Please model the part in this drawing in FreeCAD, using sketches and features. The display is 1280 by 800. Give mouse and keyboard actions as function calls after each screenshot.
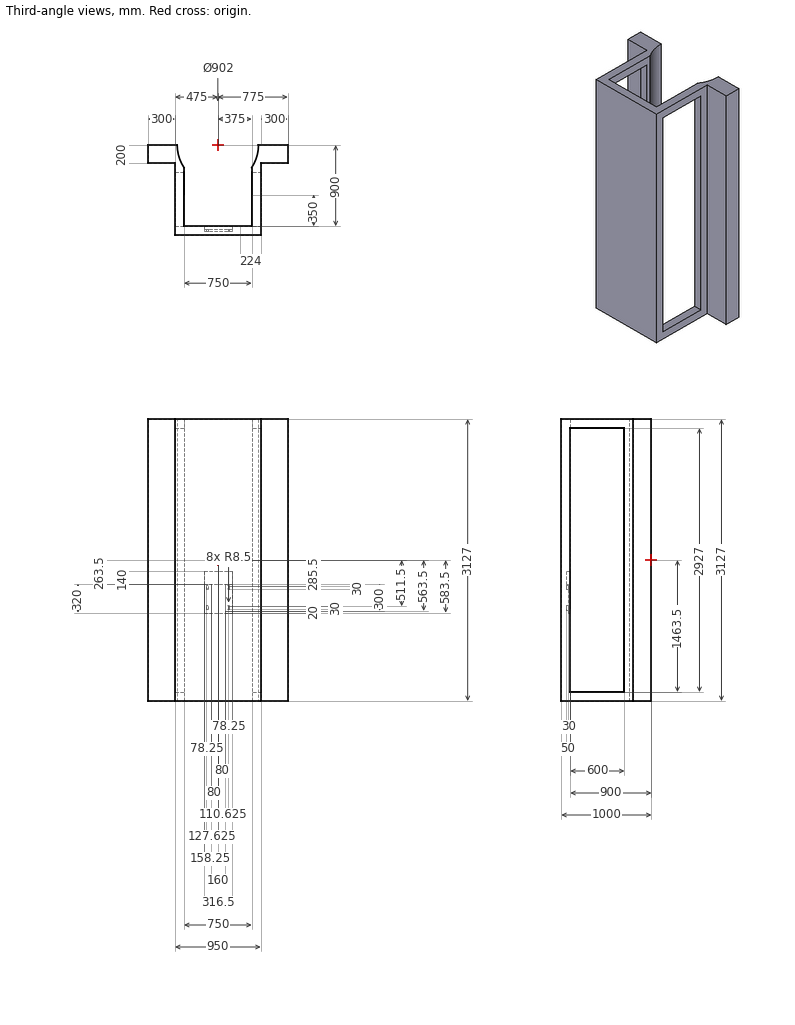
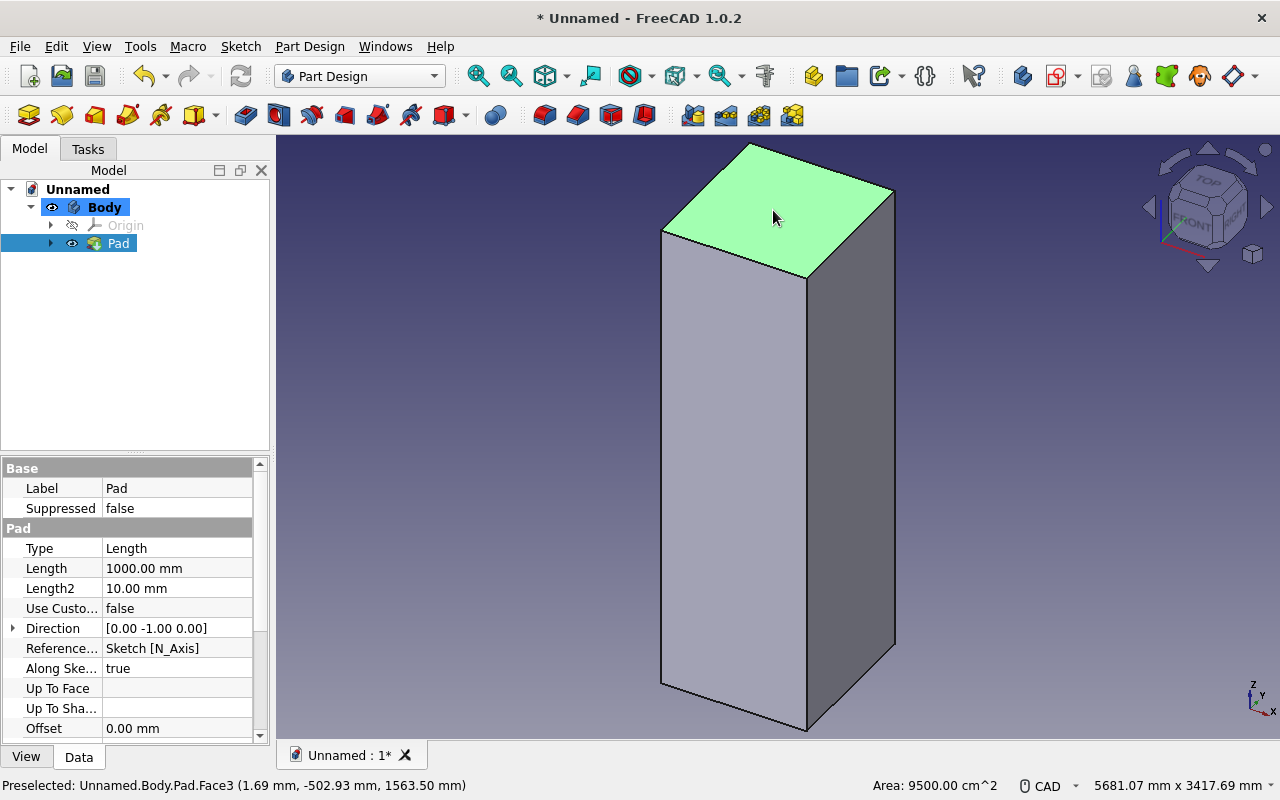
click(1056, 76)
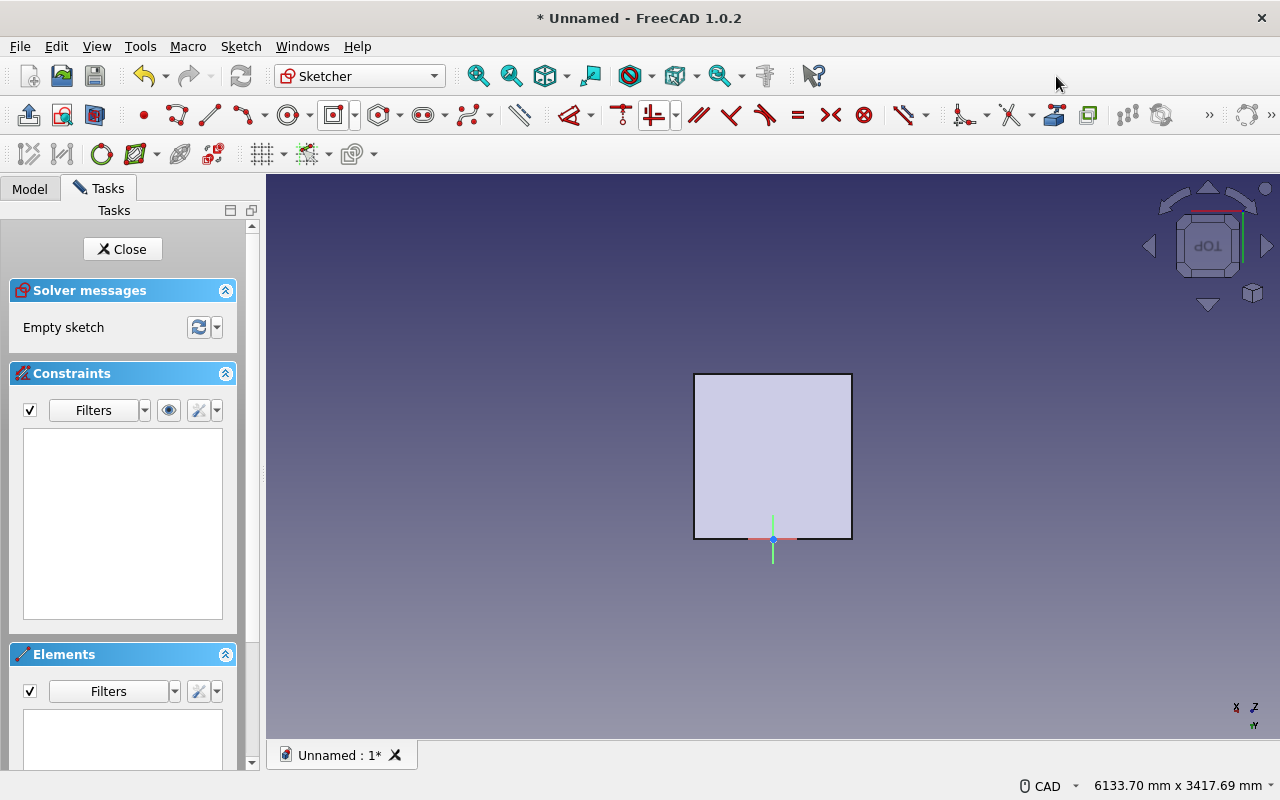
scroll(829, 607, up, 4)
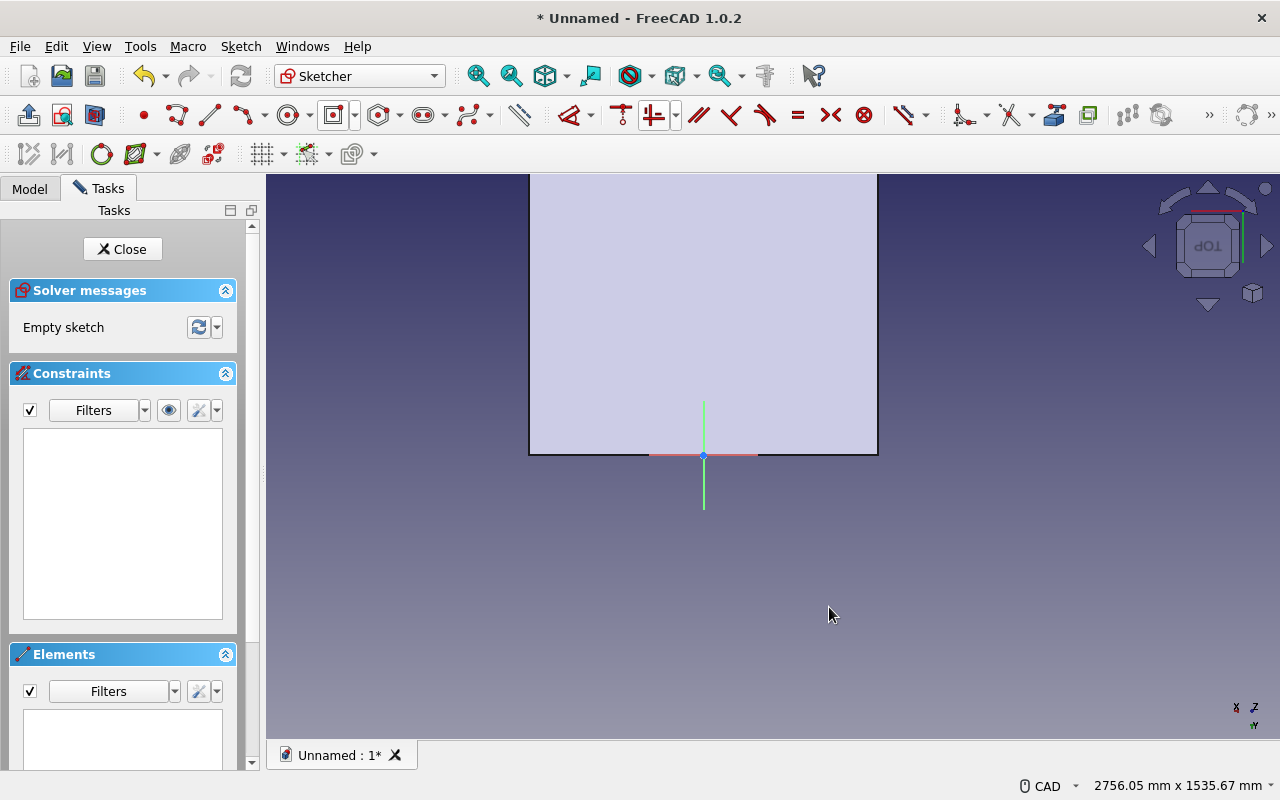
click(288, 116)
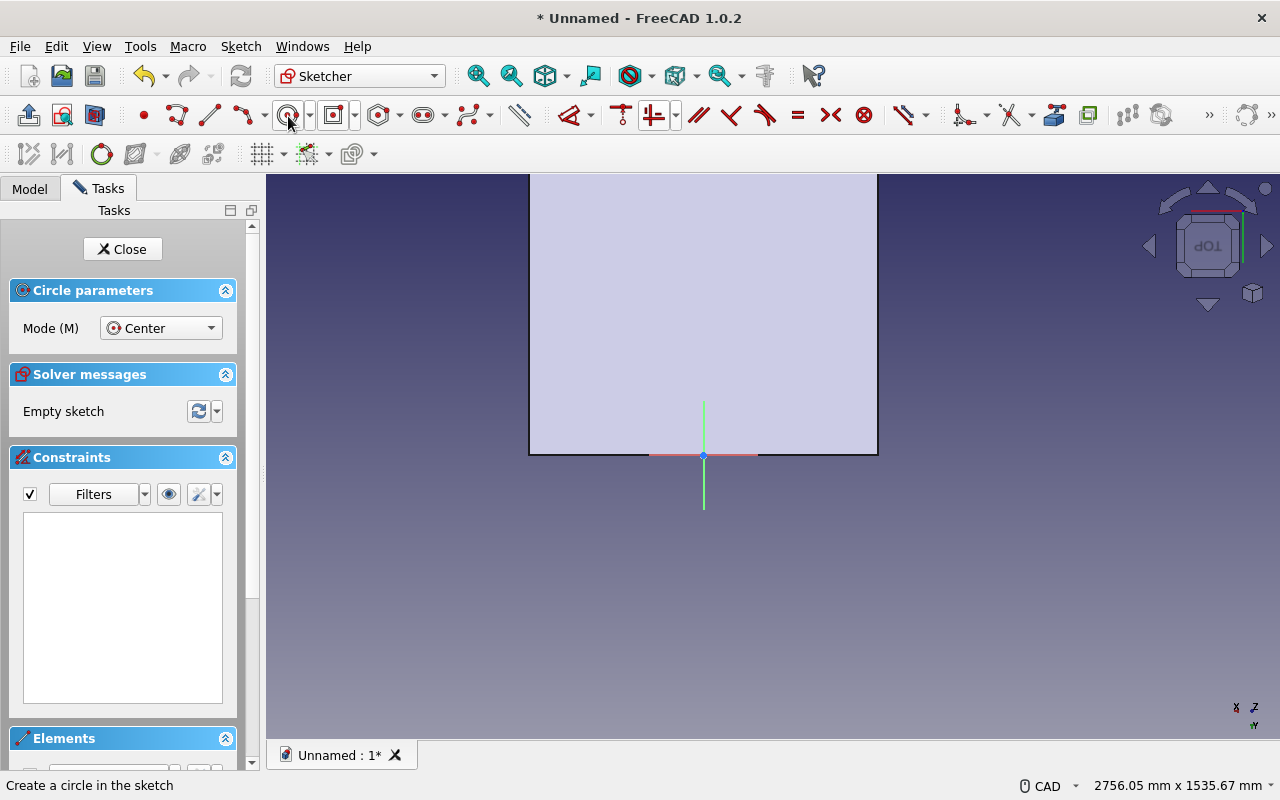
click(704, 455)
click(821, 338)
key(Escape)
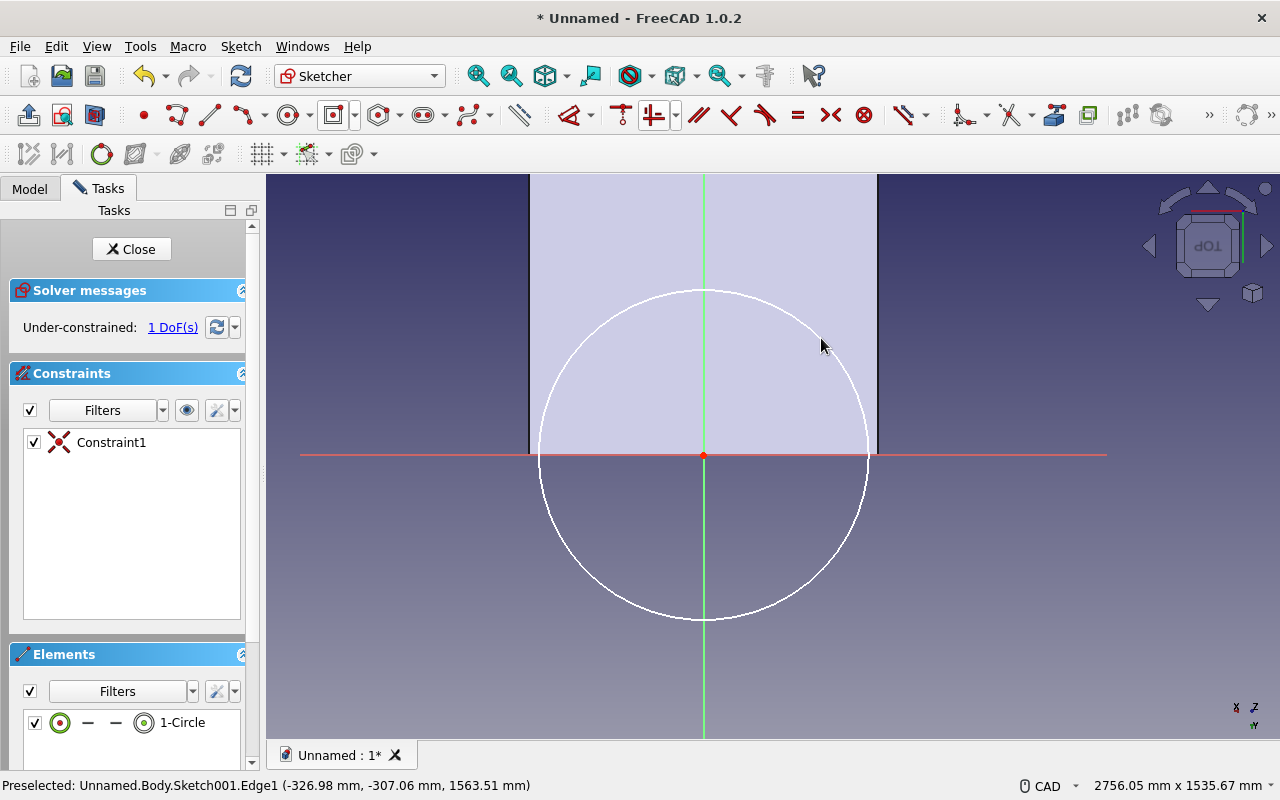
key(d)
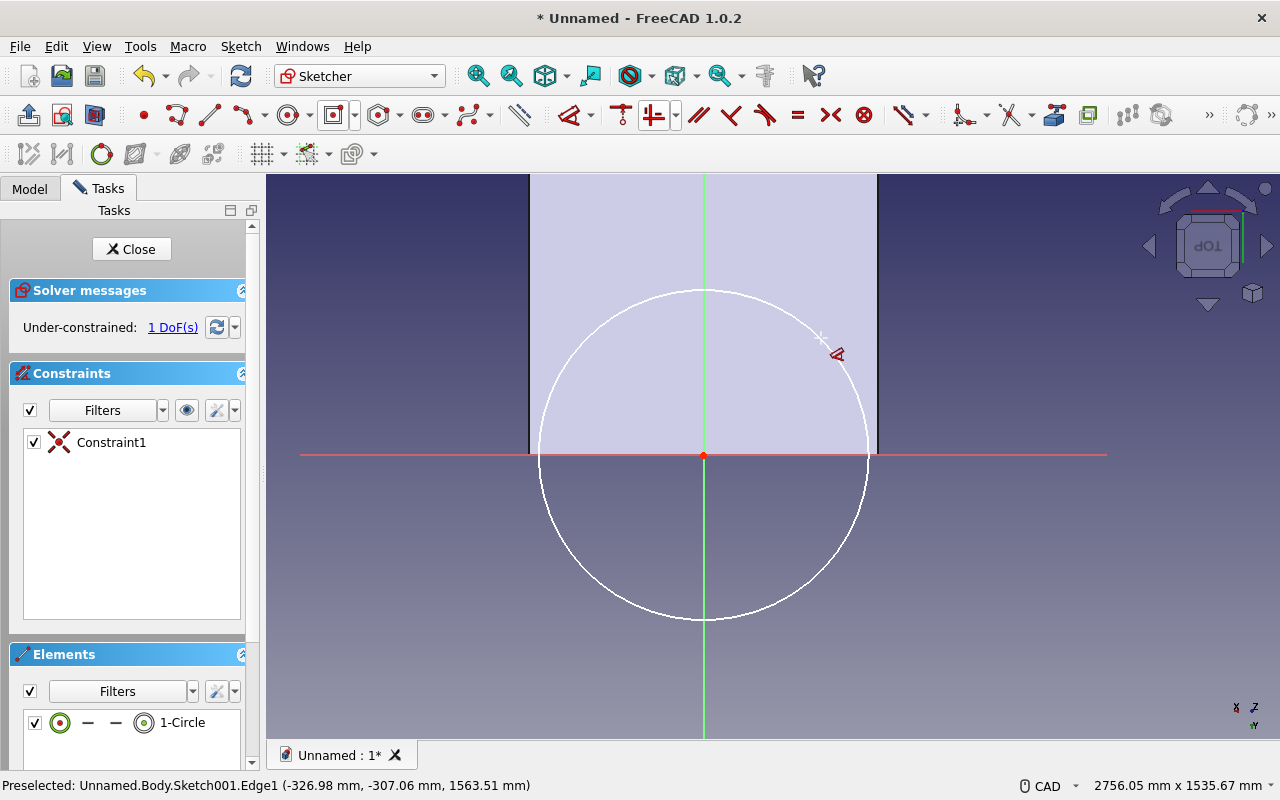
click(820, 338)
click(843, 315)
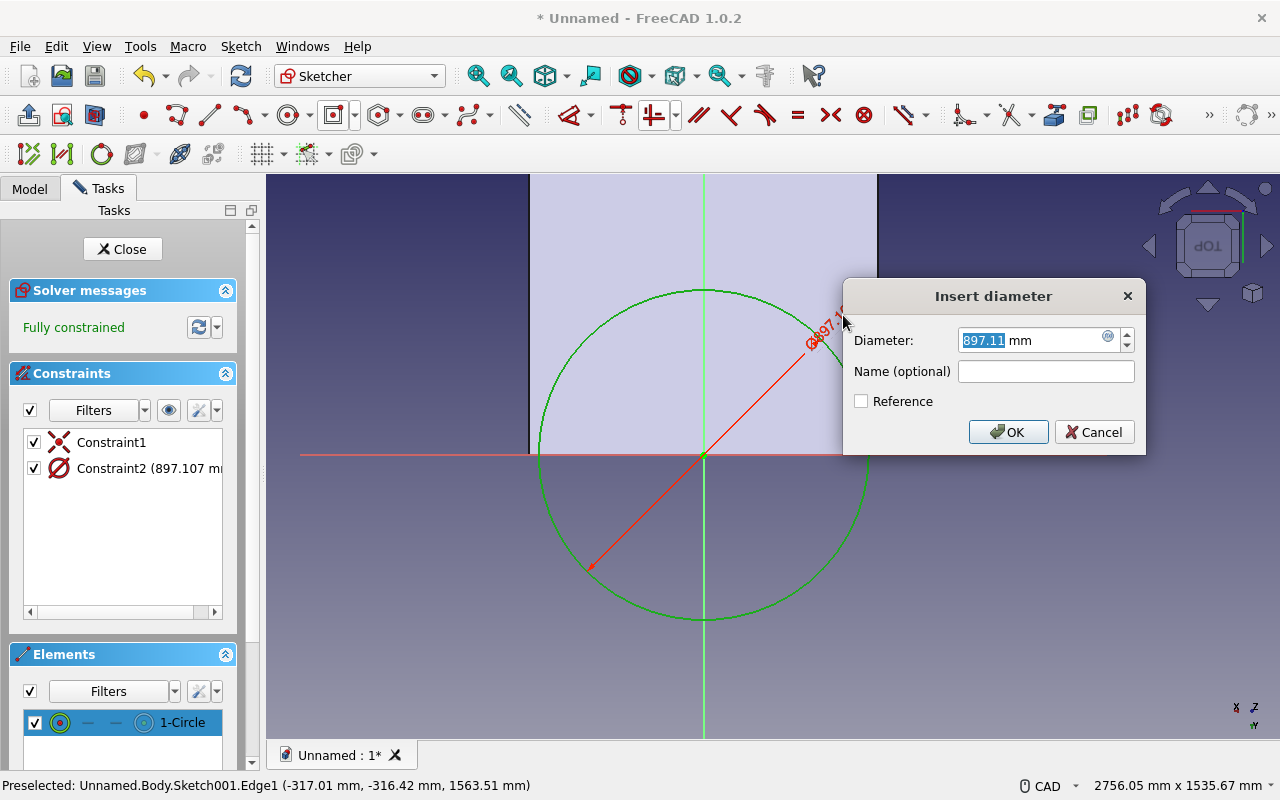
text(902)
key(Return)
key(Escape)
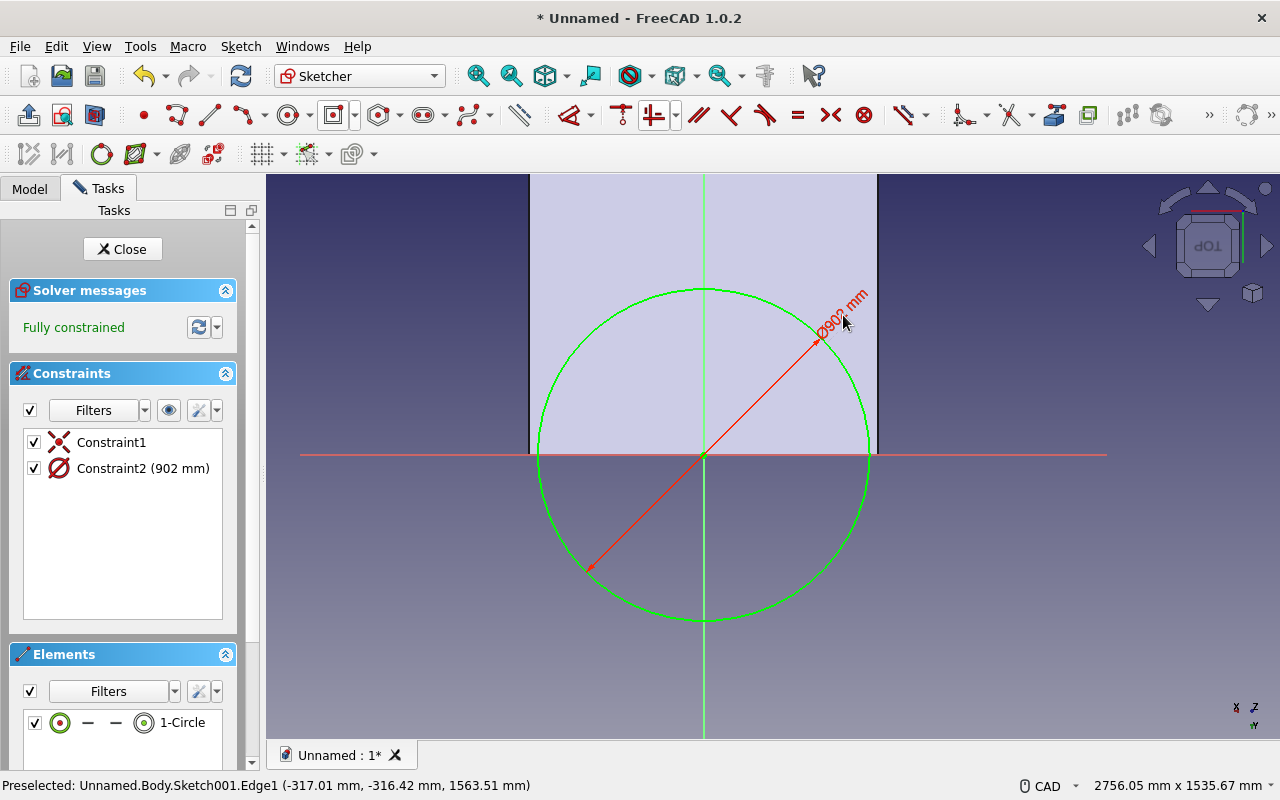
click(123, 249)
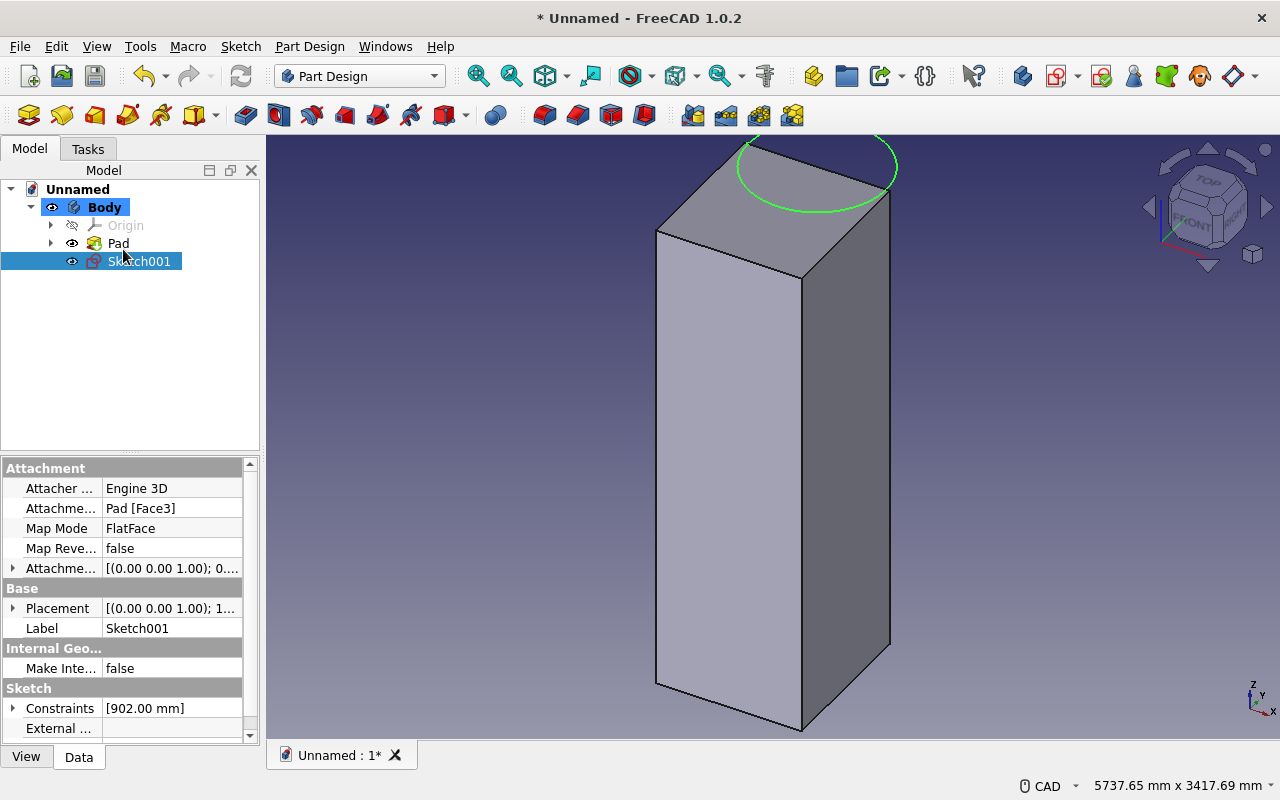
click(246, 116)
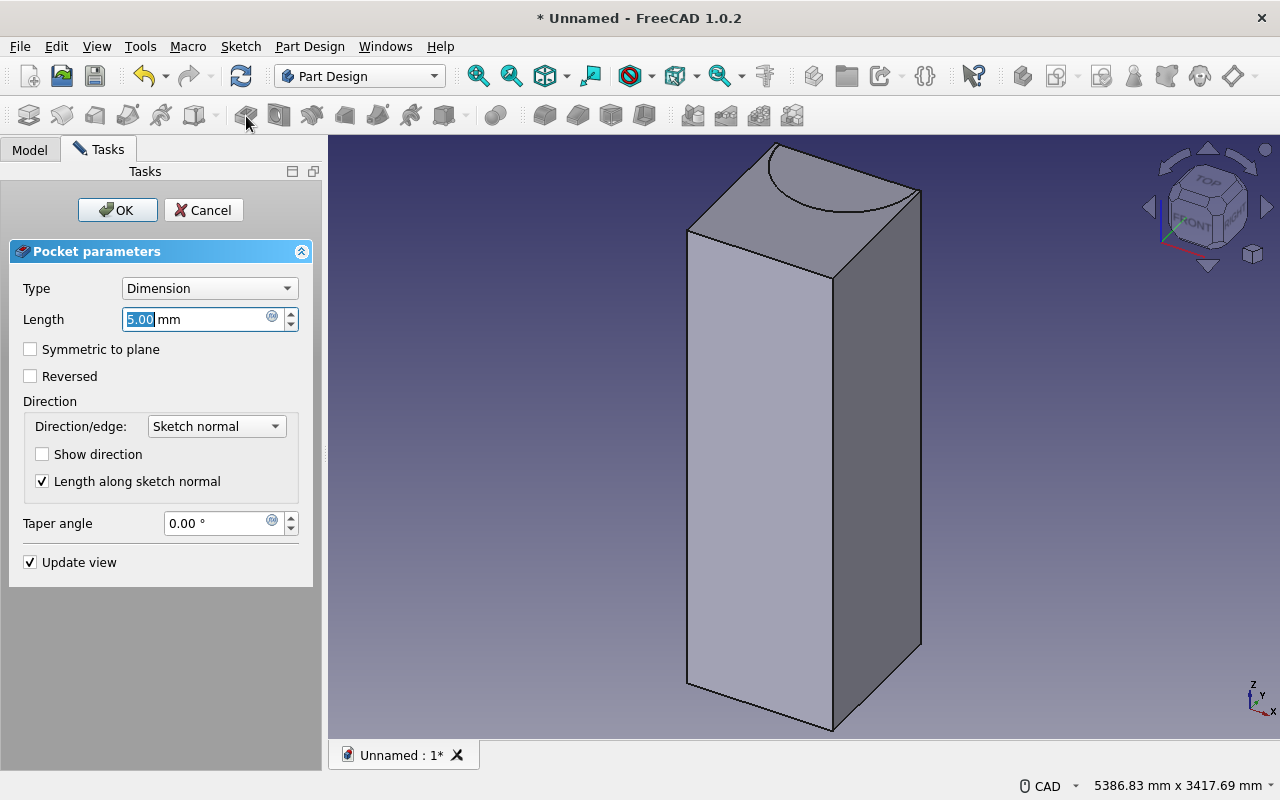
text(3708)
key(Tab)